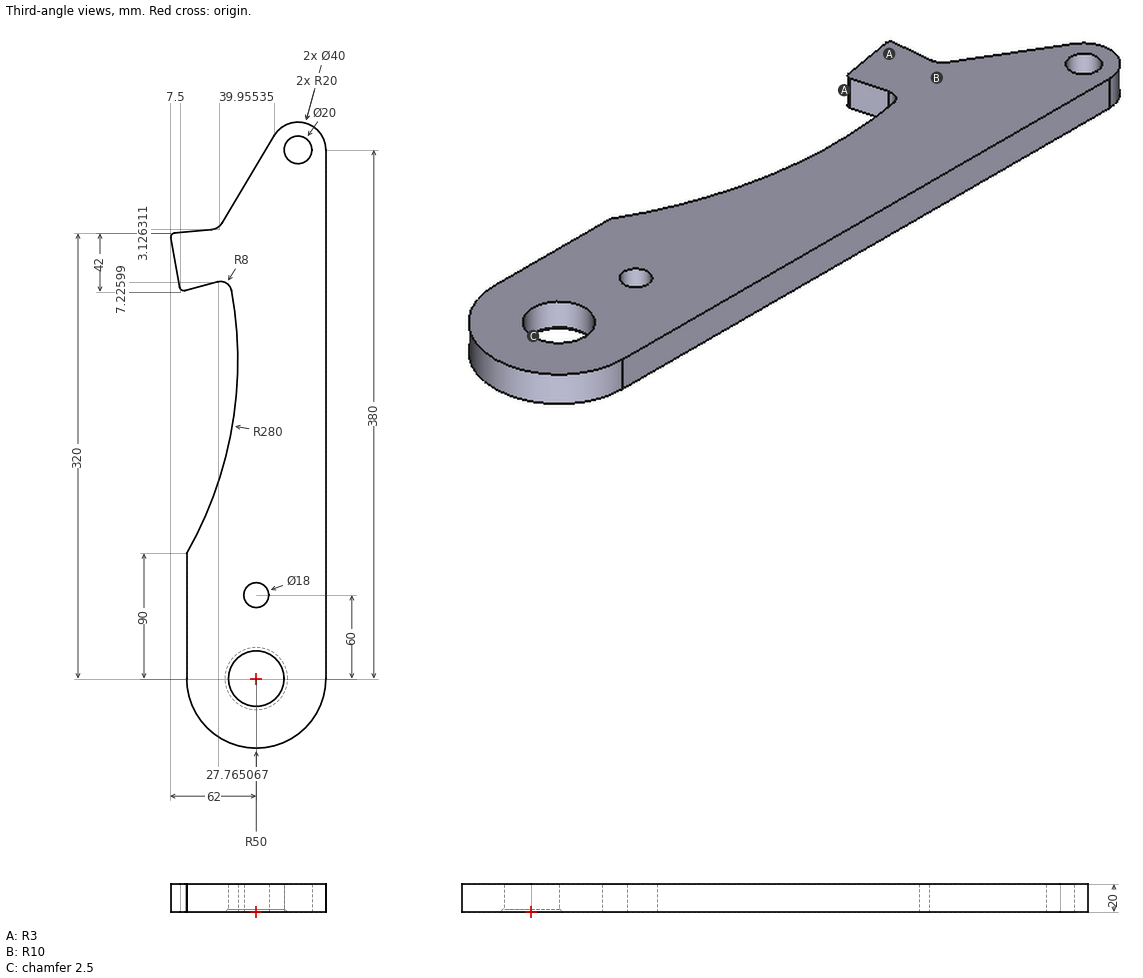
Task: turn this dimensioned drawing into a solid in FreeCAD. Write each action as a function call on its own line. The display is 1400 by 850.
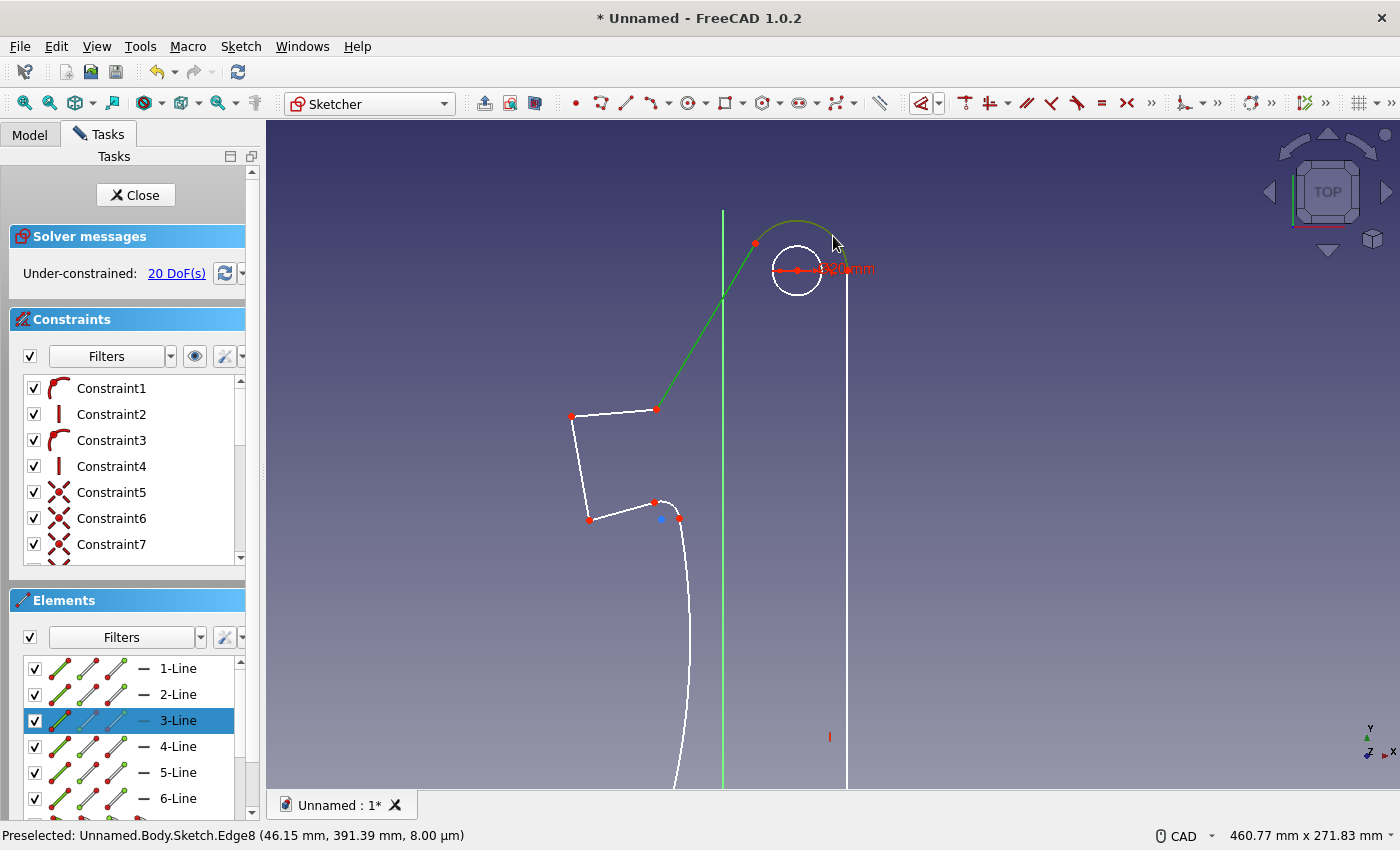
click(1077, 104)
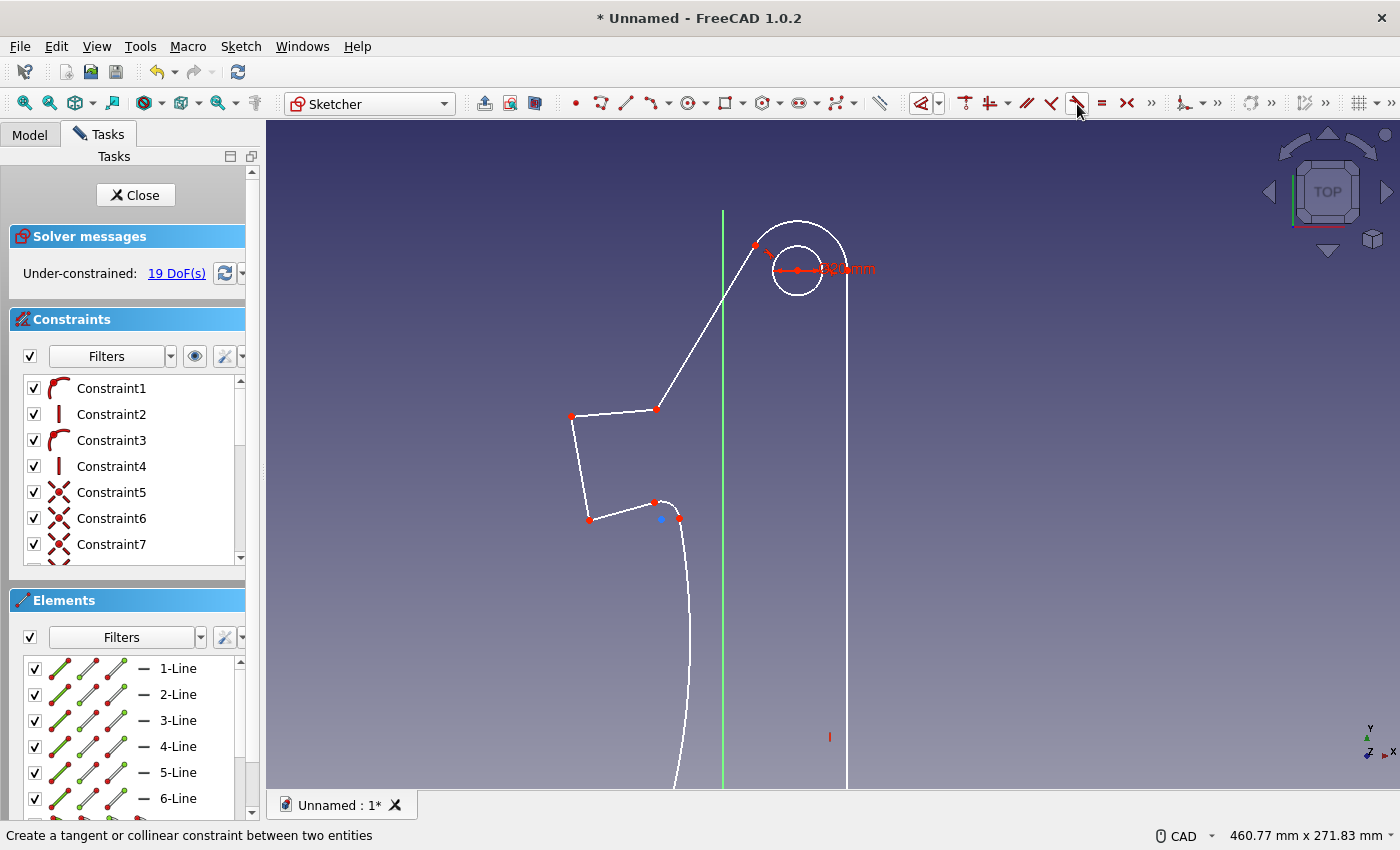
click(609, 515)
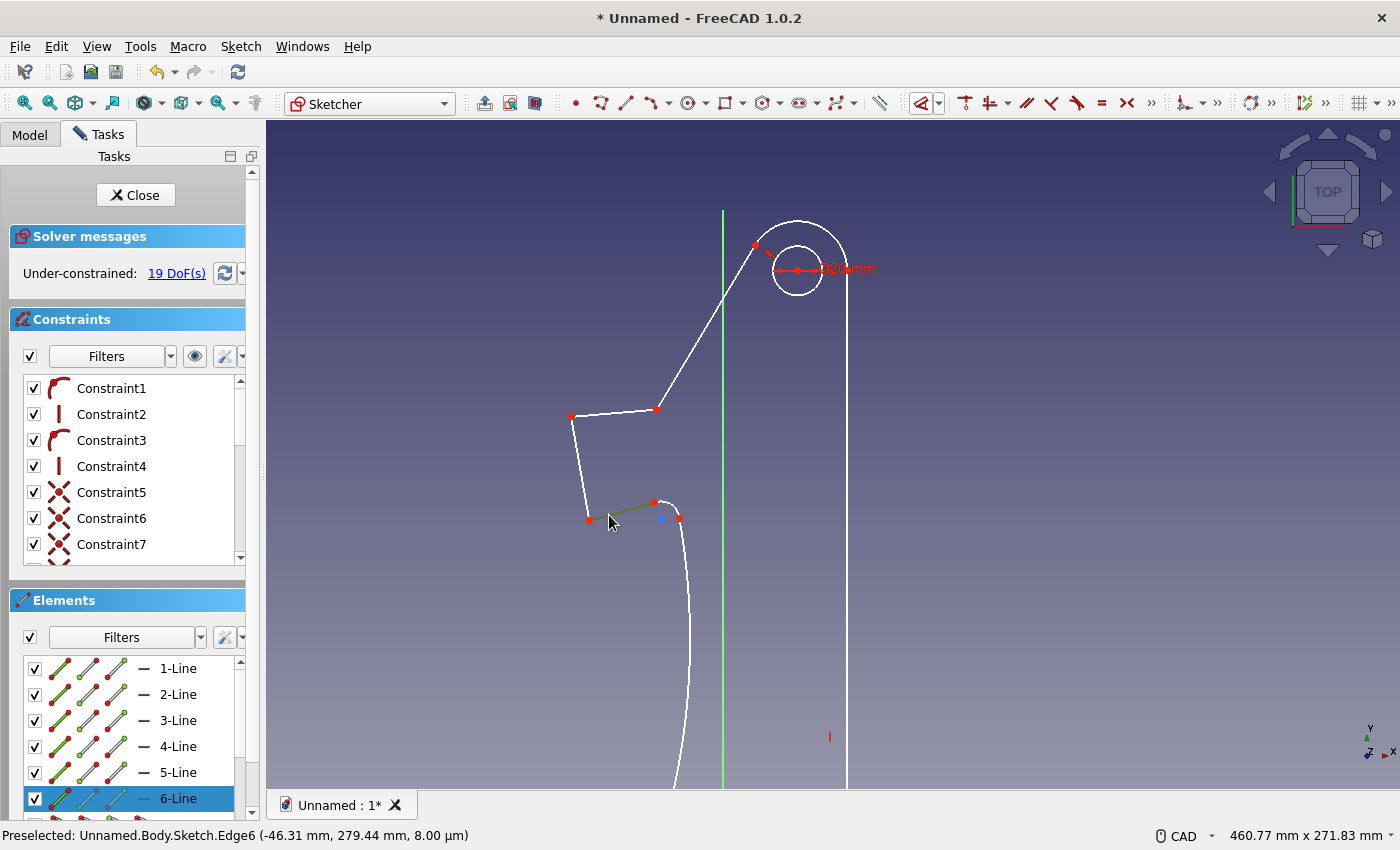
scroll(676, 509, up, 2)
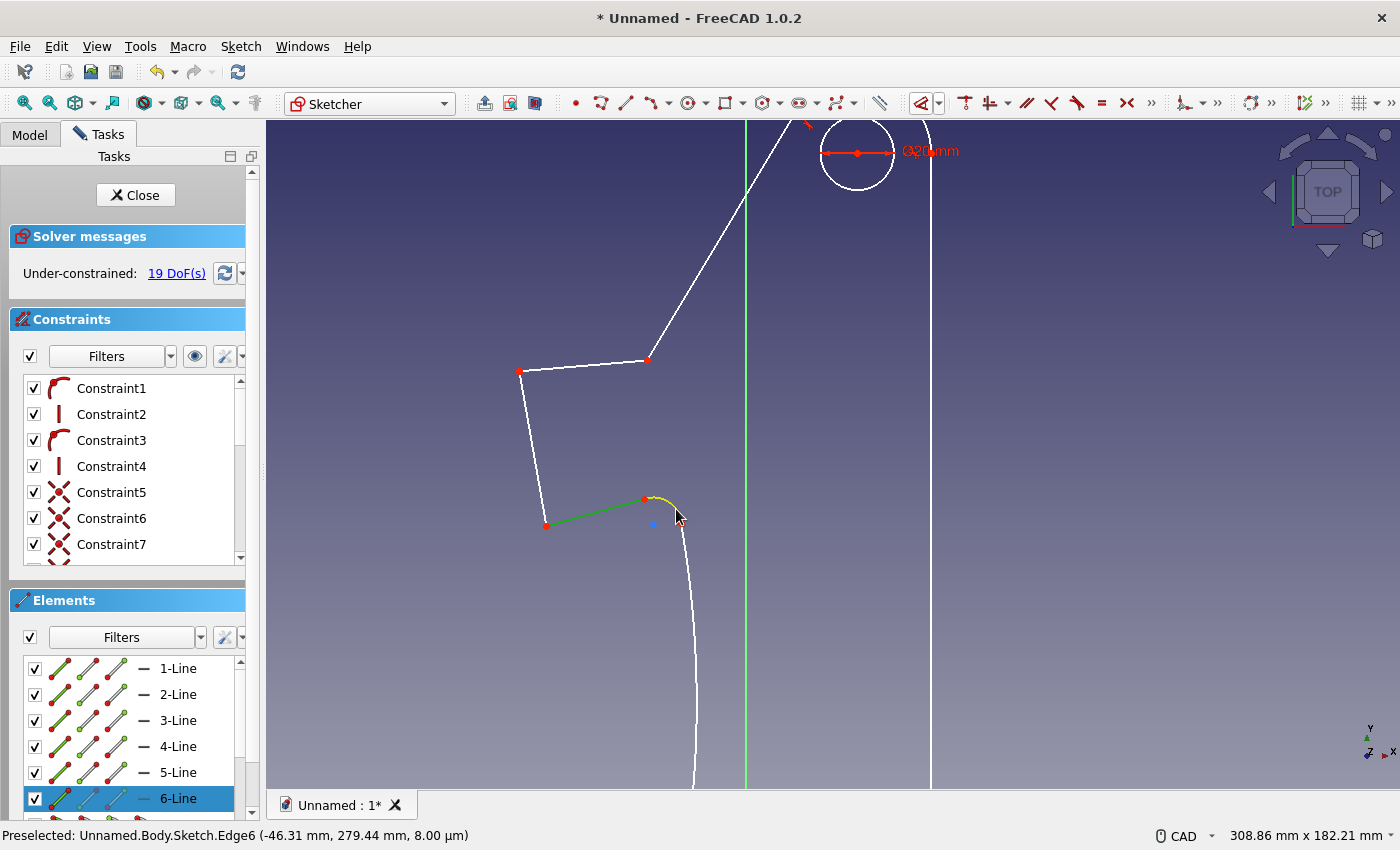
click(676, 509)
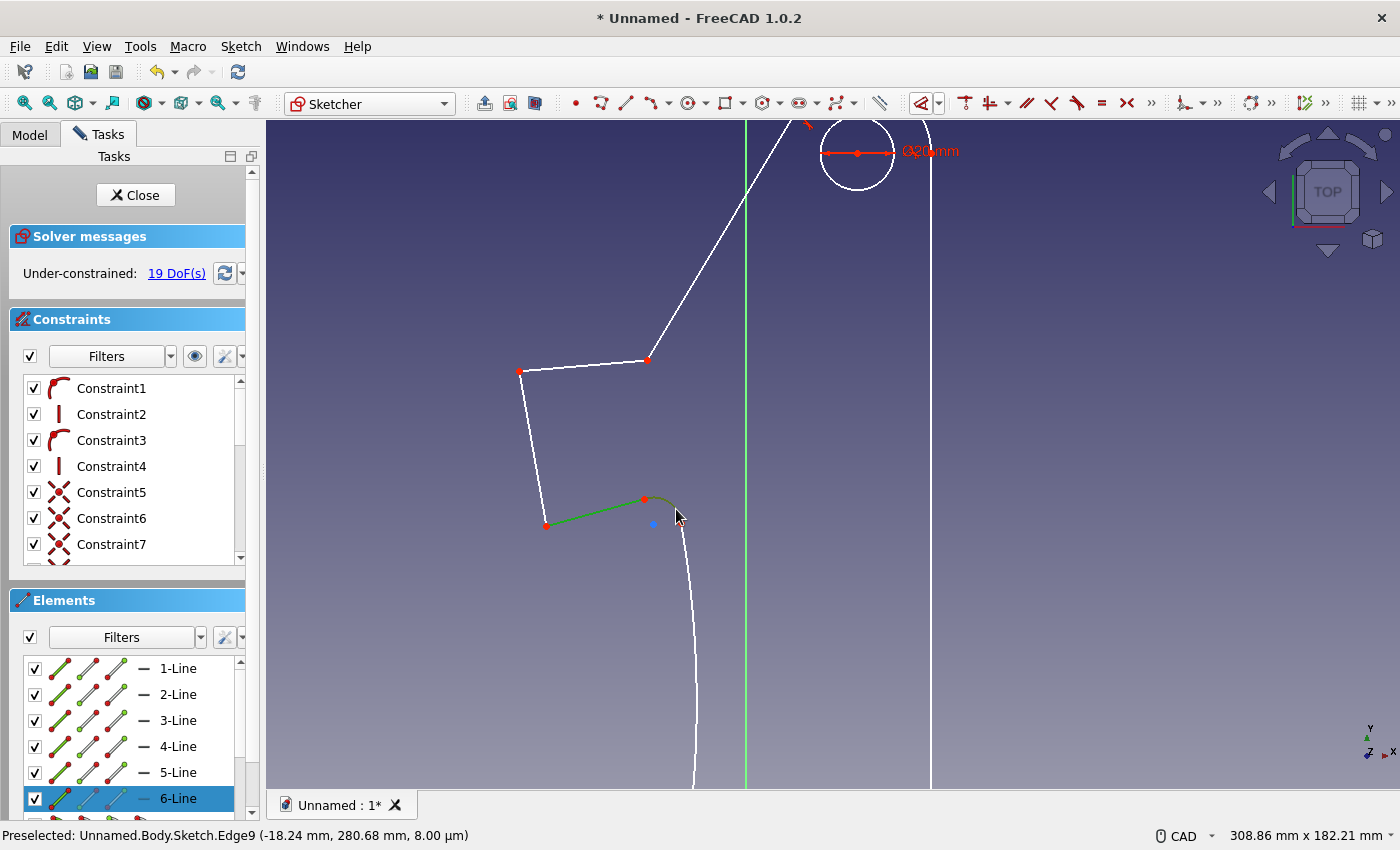
click(1077, 104)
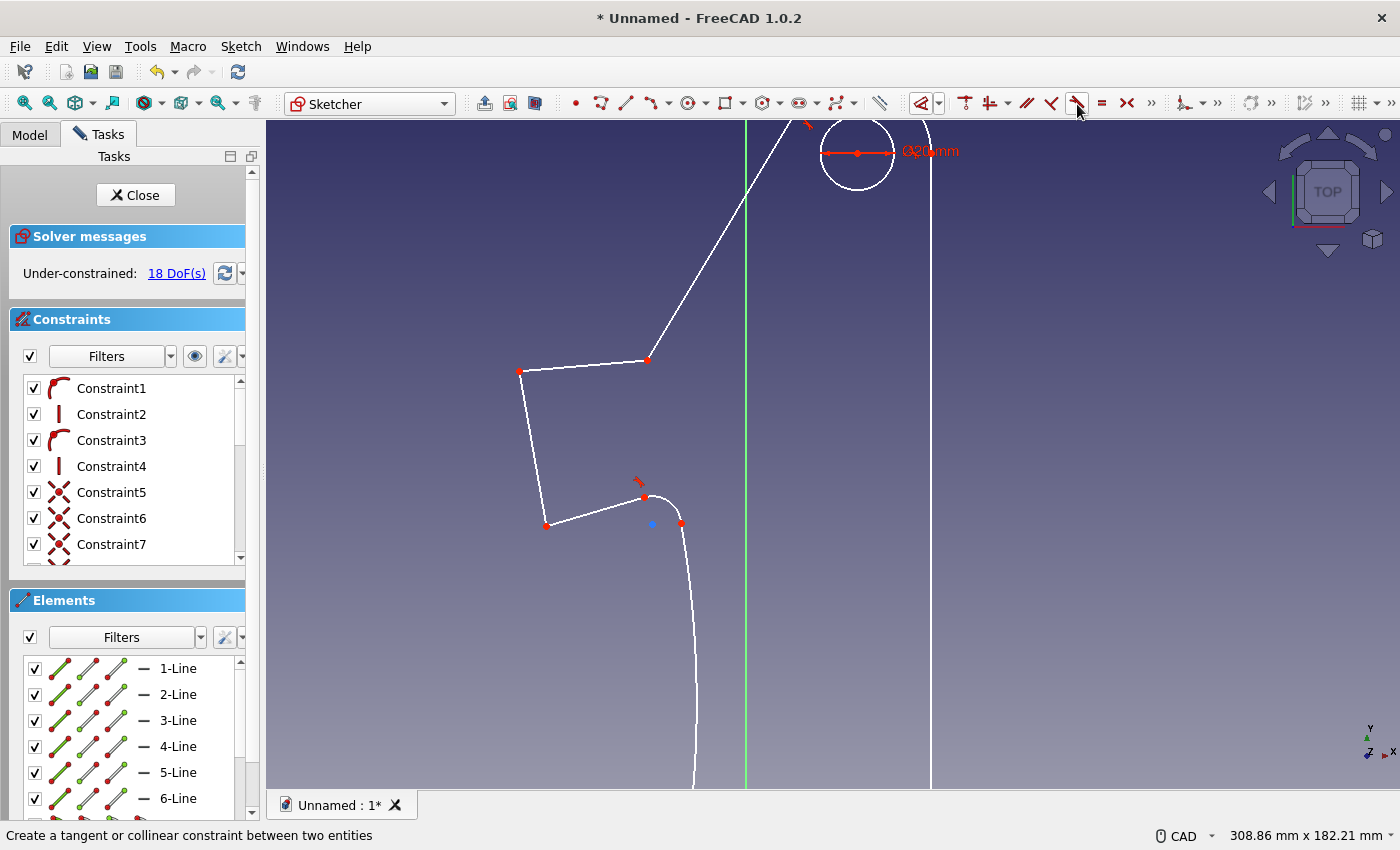
click(676, 509)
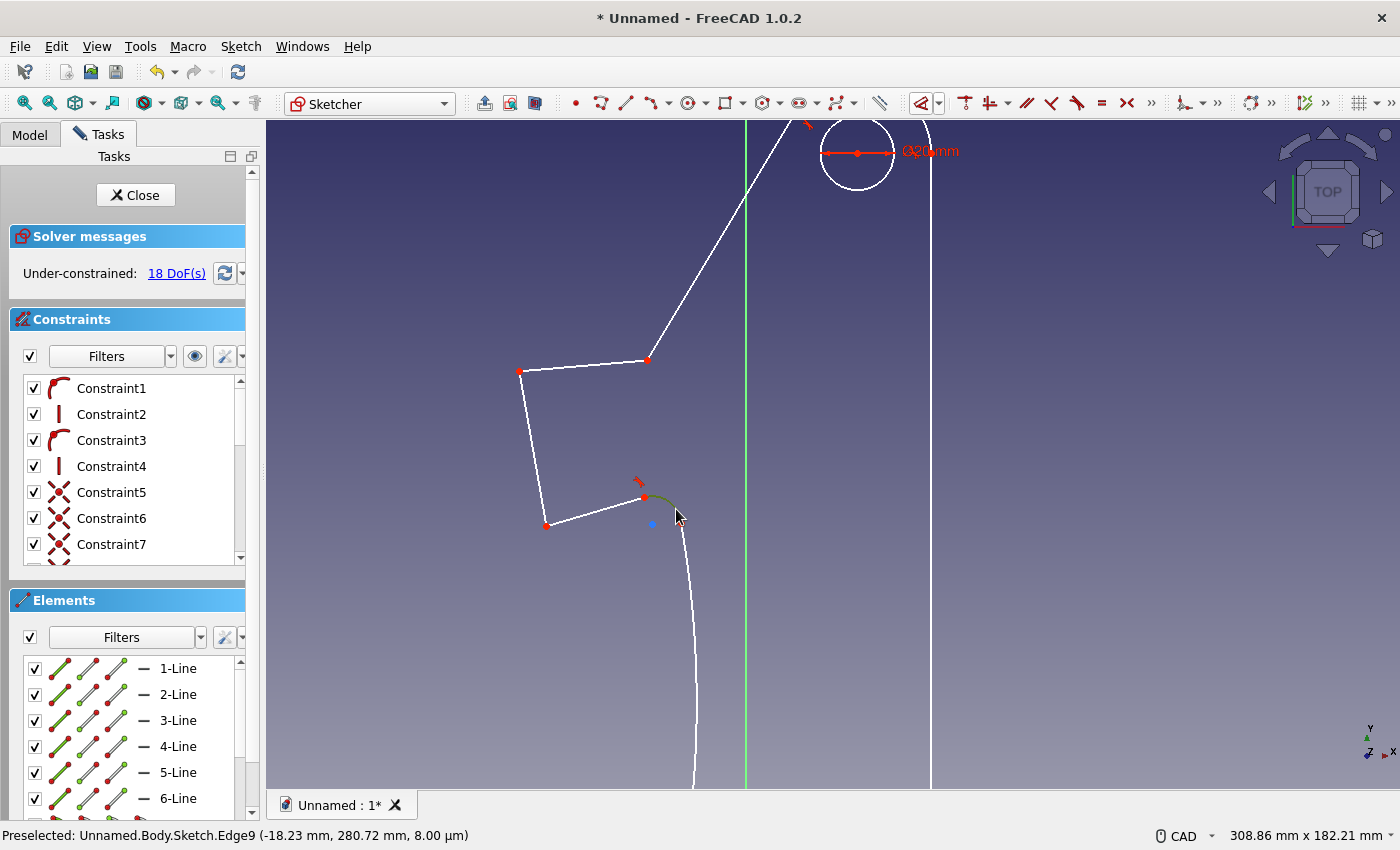
scroll(778, 308, down, 7)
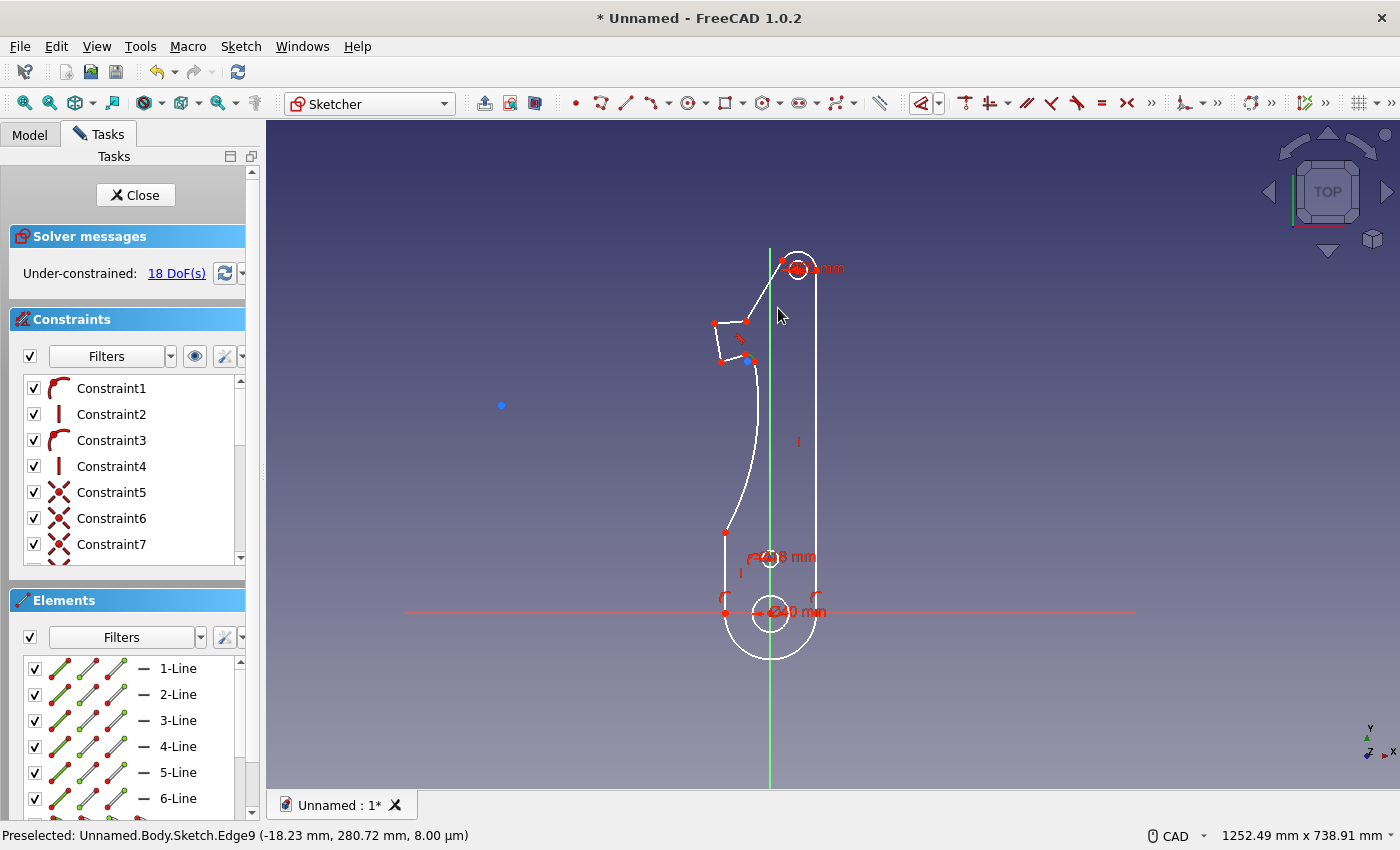
click(758, 414)